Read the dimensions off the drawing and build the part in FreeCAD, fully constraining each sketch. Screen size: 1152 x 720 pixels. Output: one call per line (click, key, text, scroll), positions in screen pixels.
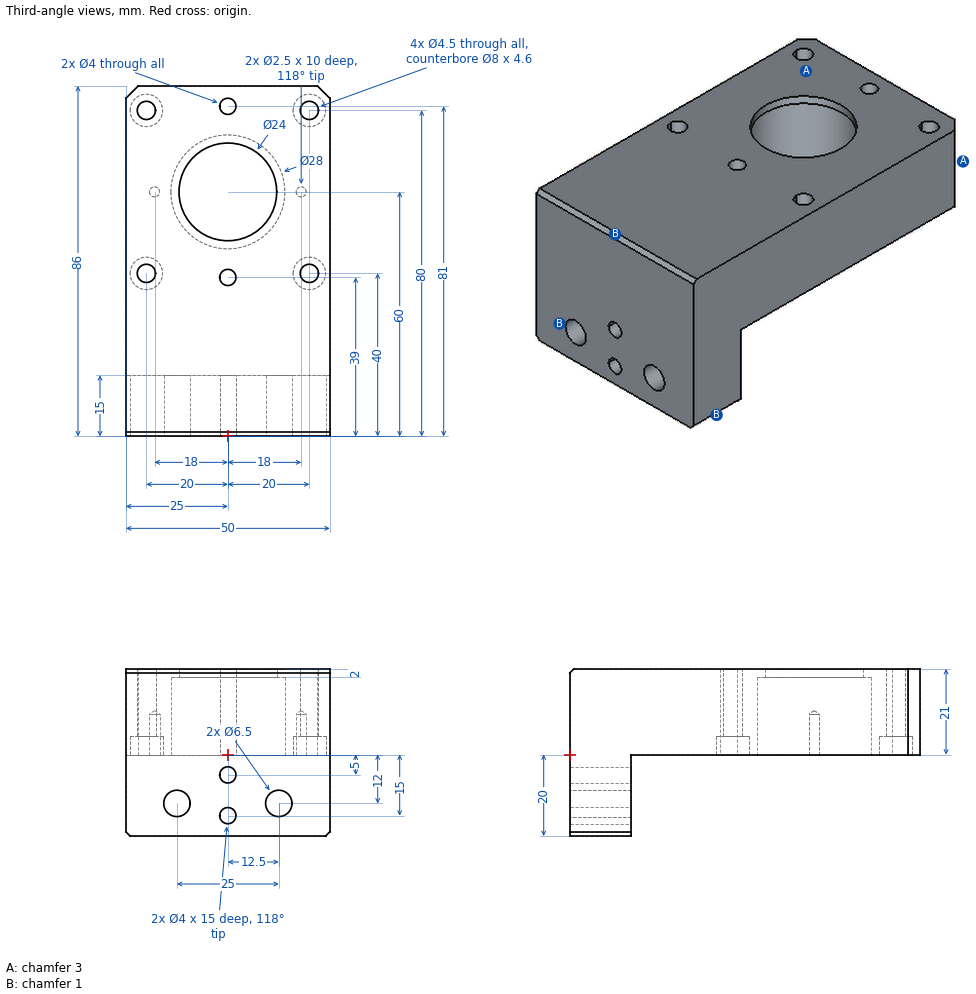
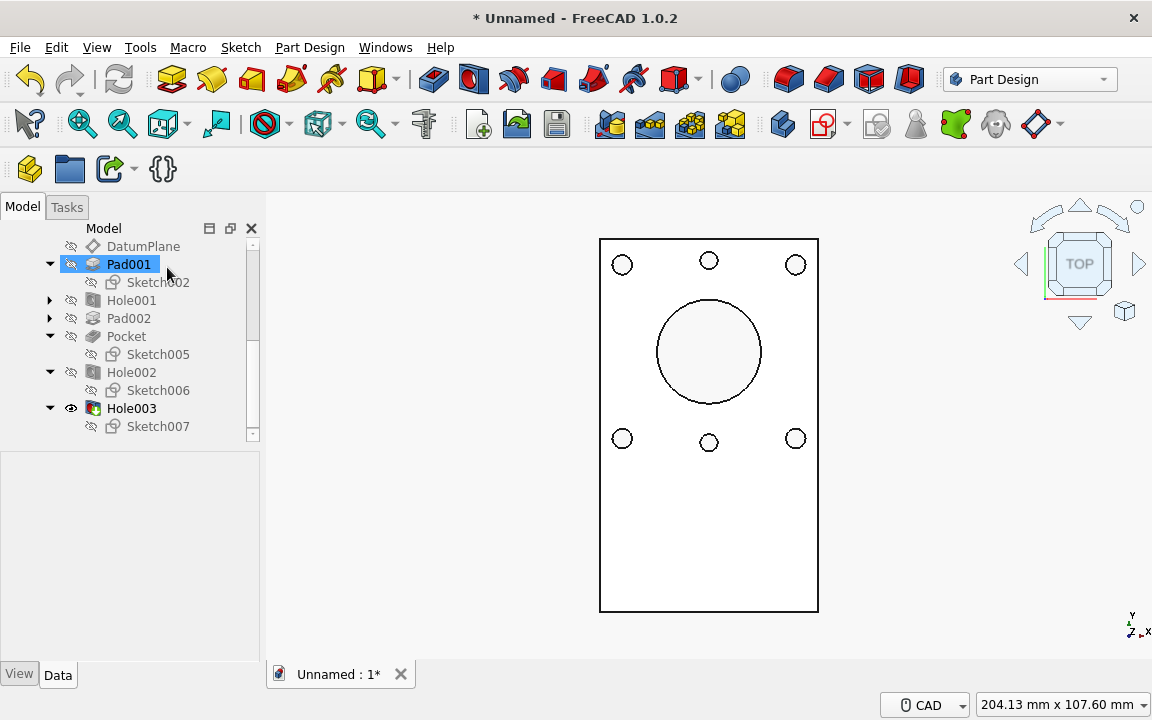
key(0)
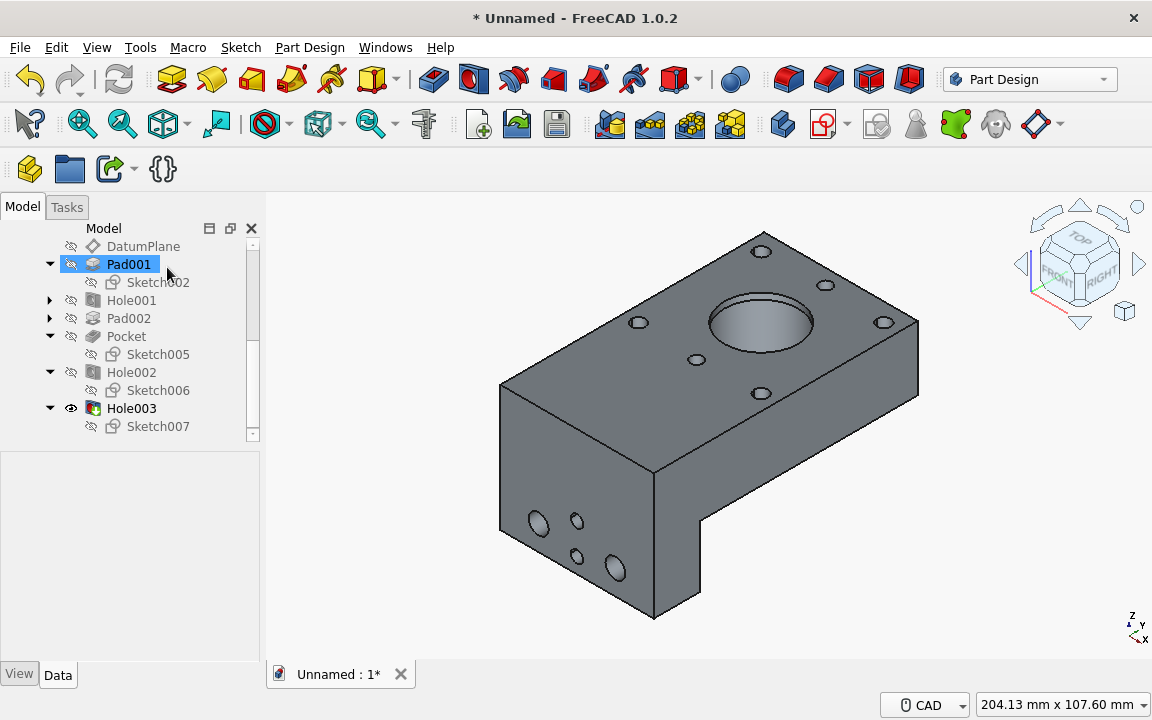
key(1)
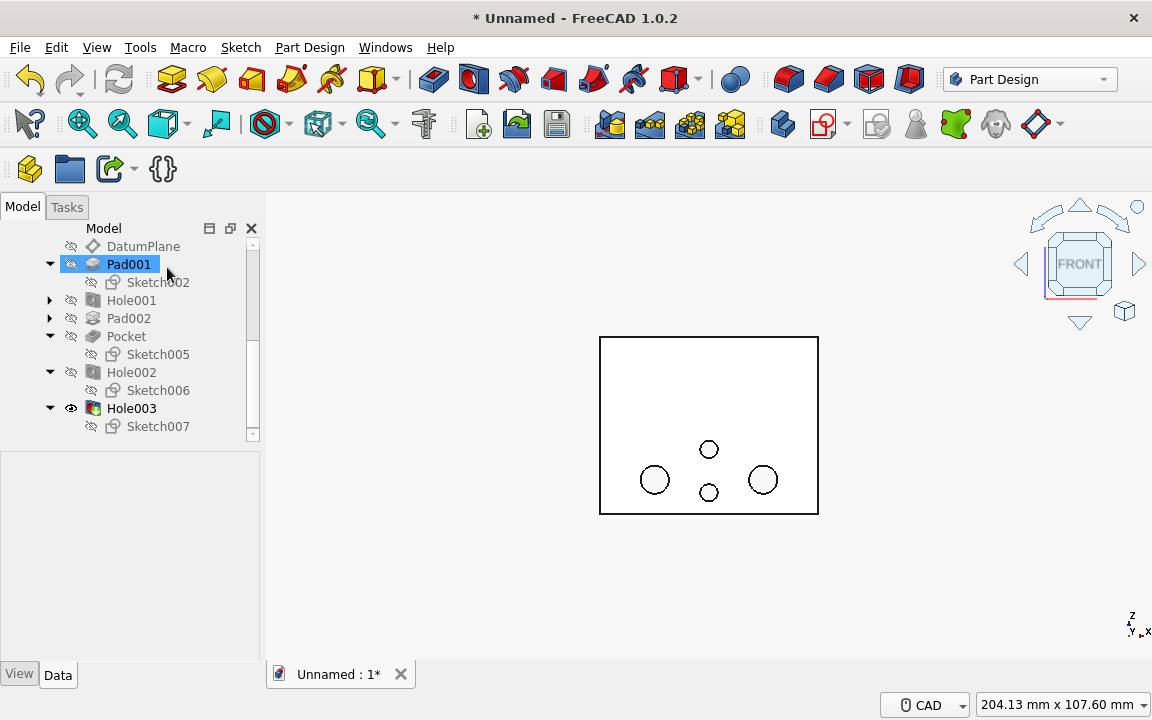
click(84, 124)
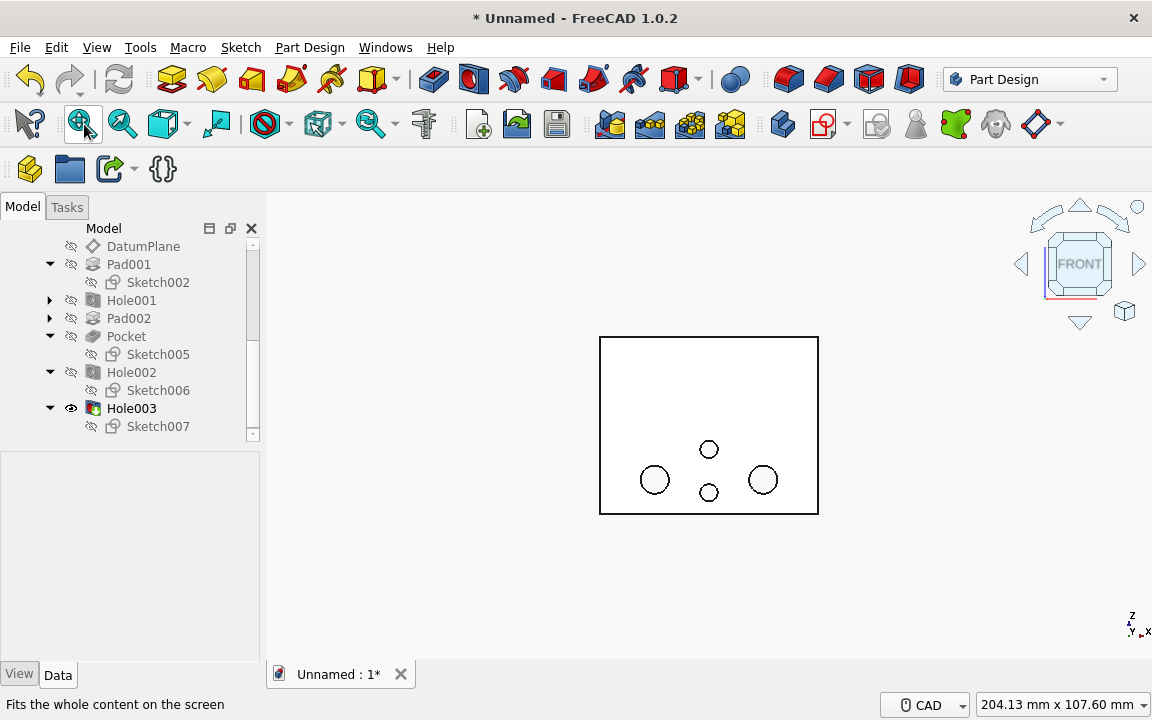
key(3)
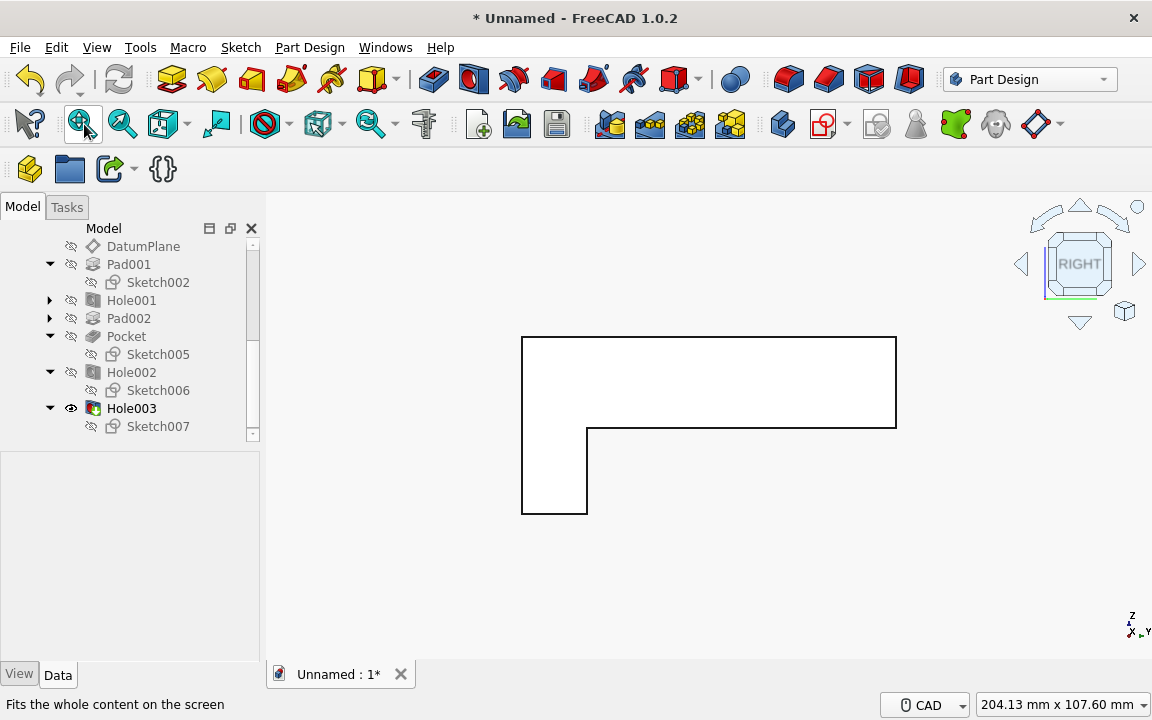
click(84, 124)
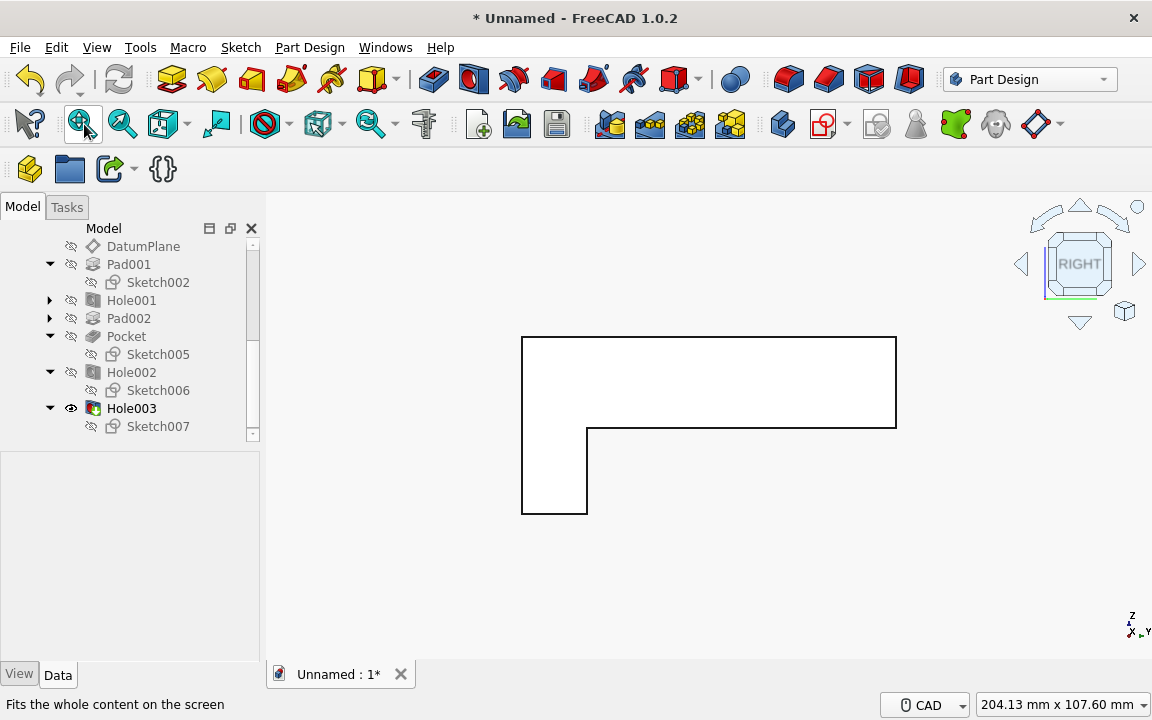
click(896, 381)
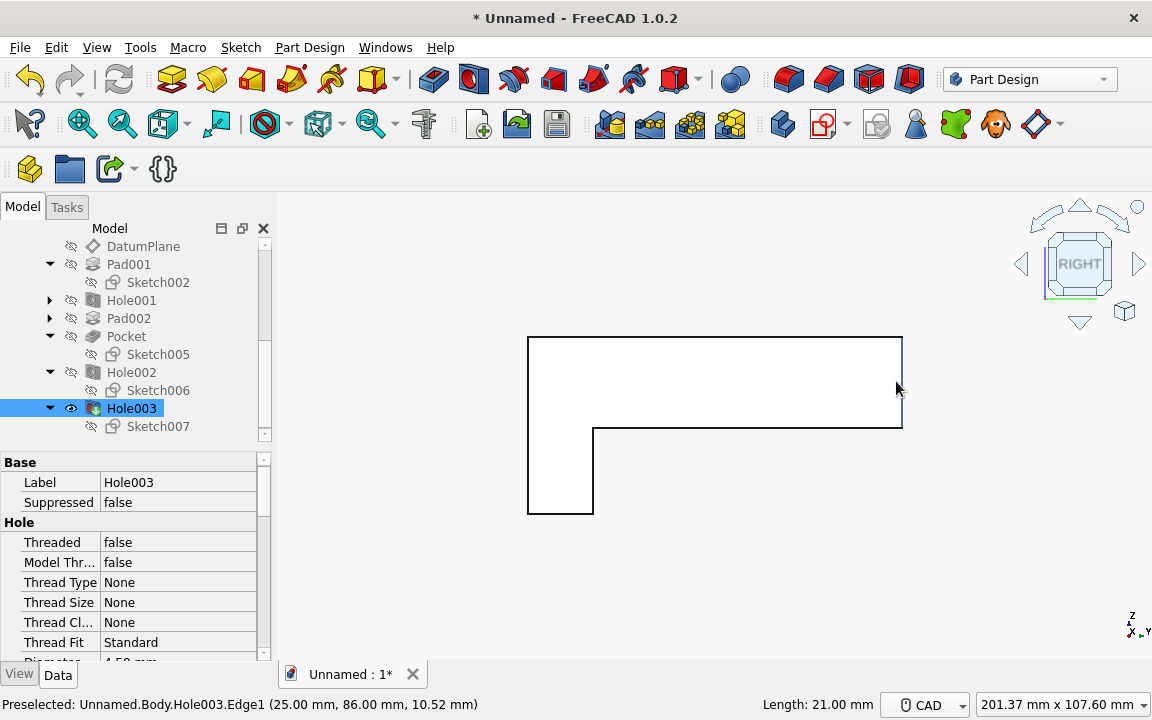
key(5)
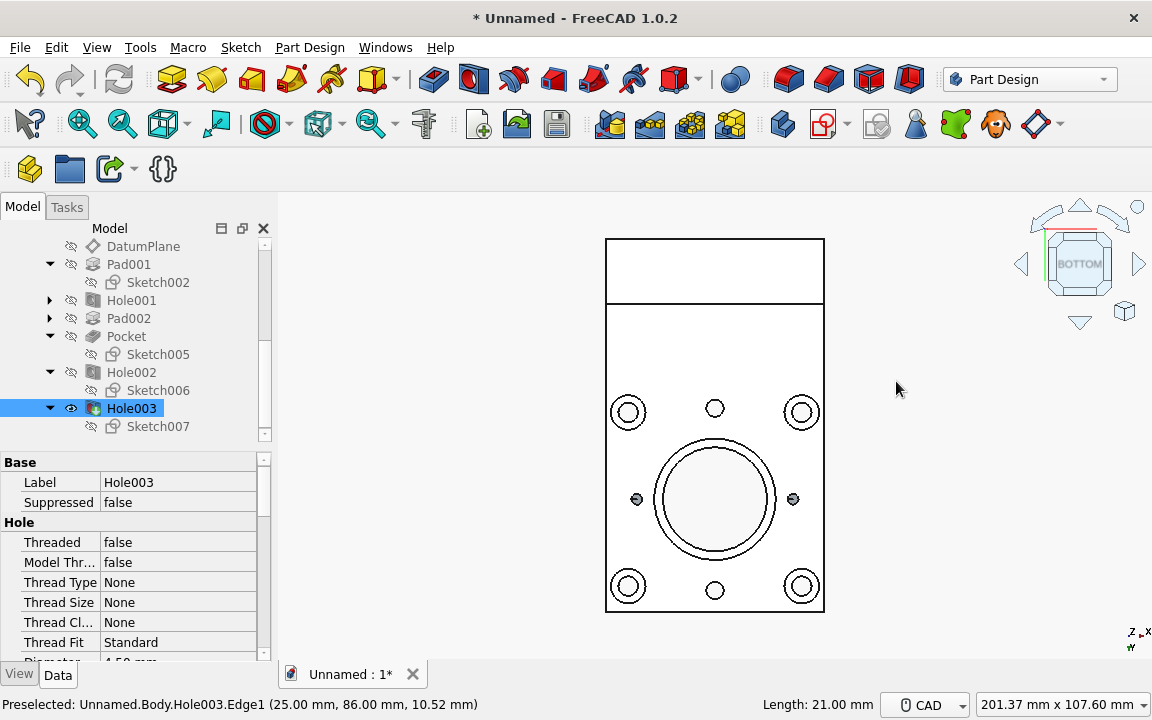
key(4)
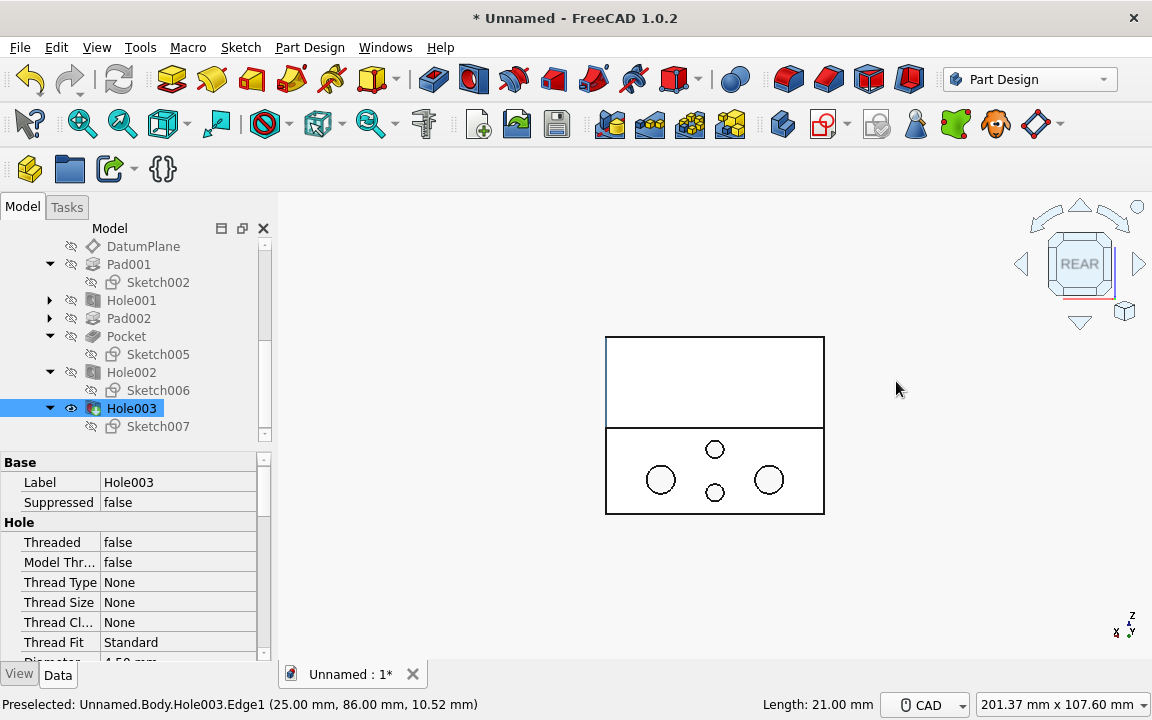
click(84, 124)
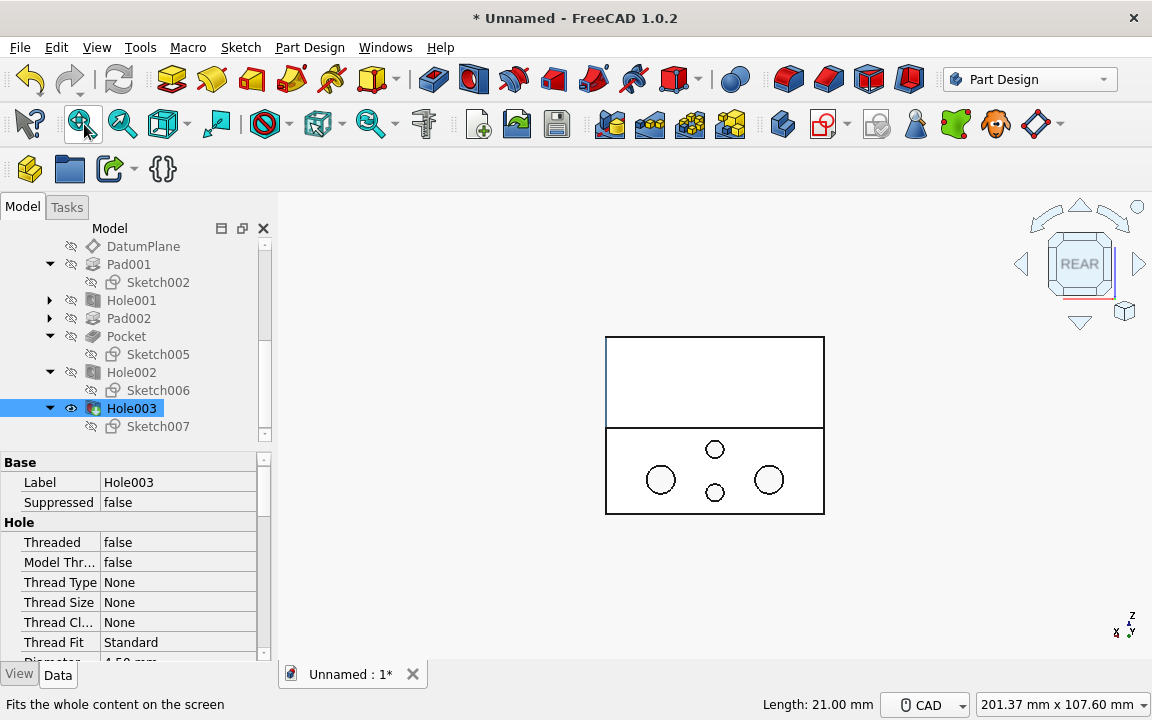
click(824, 381, ctrl)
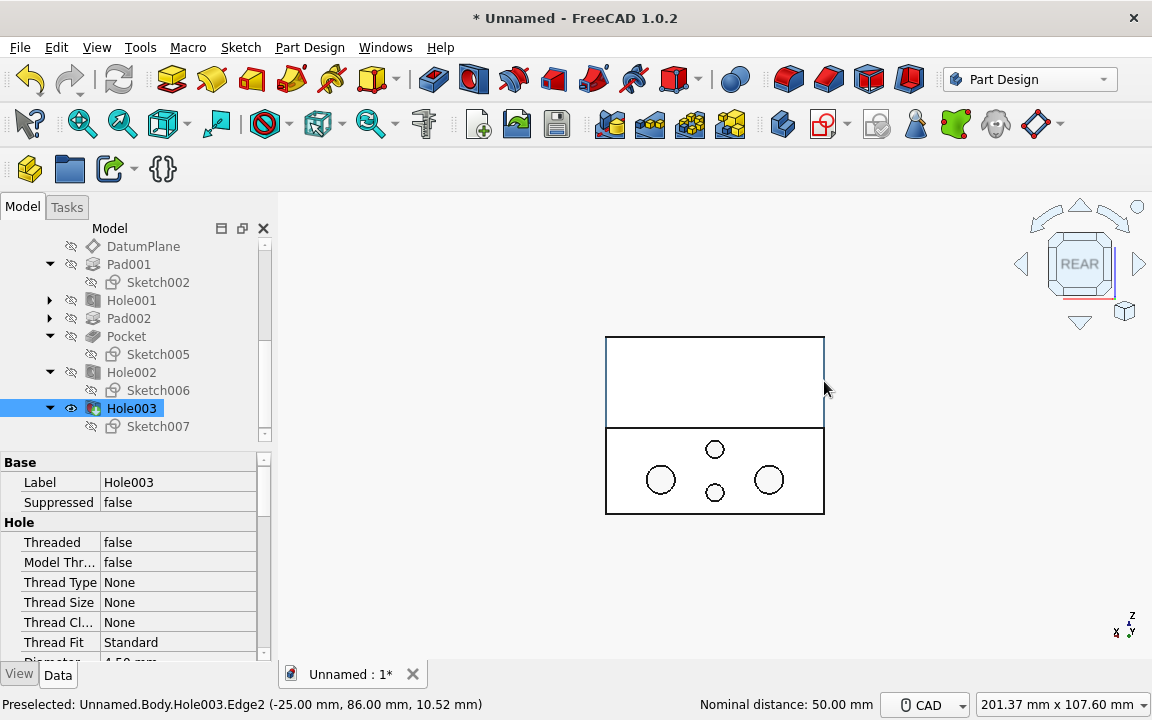
click(830, 80)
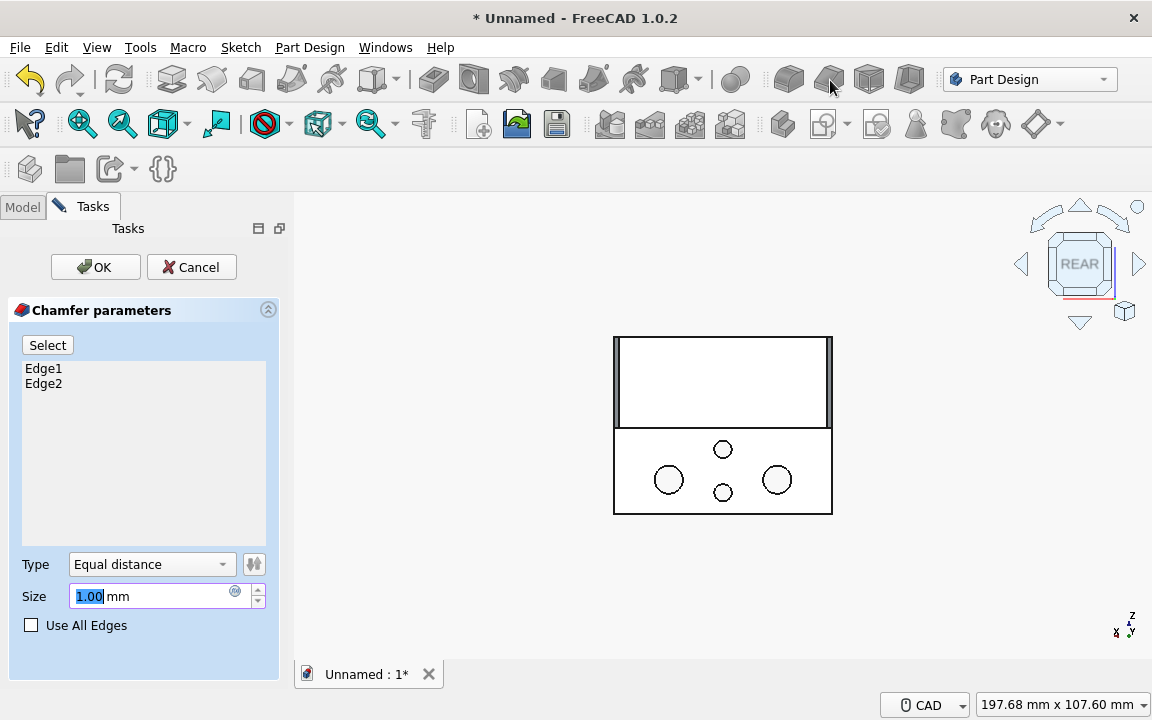
text(3)
key(Tab)